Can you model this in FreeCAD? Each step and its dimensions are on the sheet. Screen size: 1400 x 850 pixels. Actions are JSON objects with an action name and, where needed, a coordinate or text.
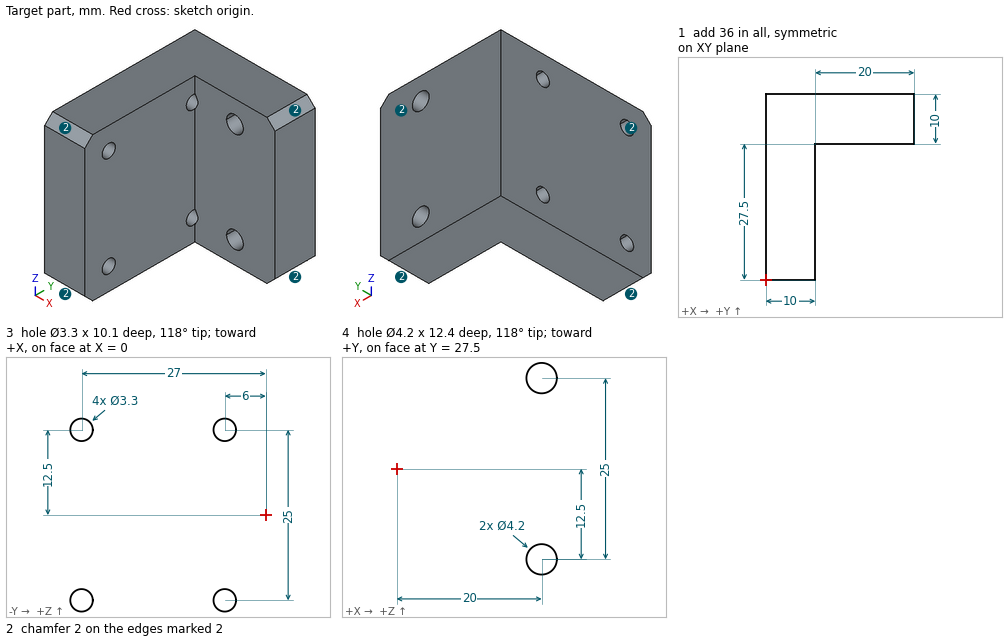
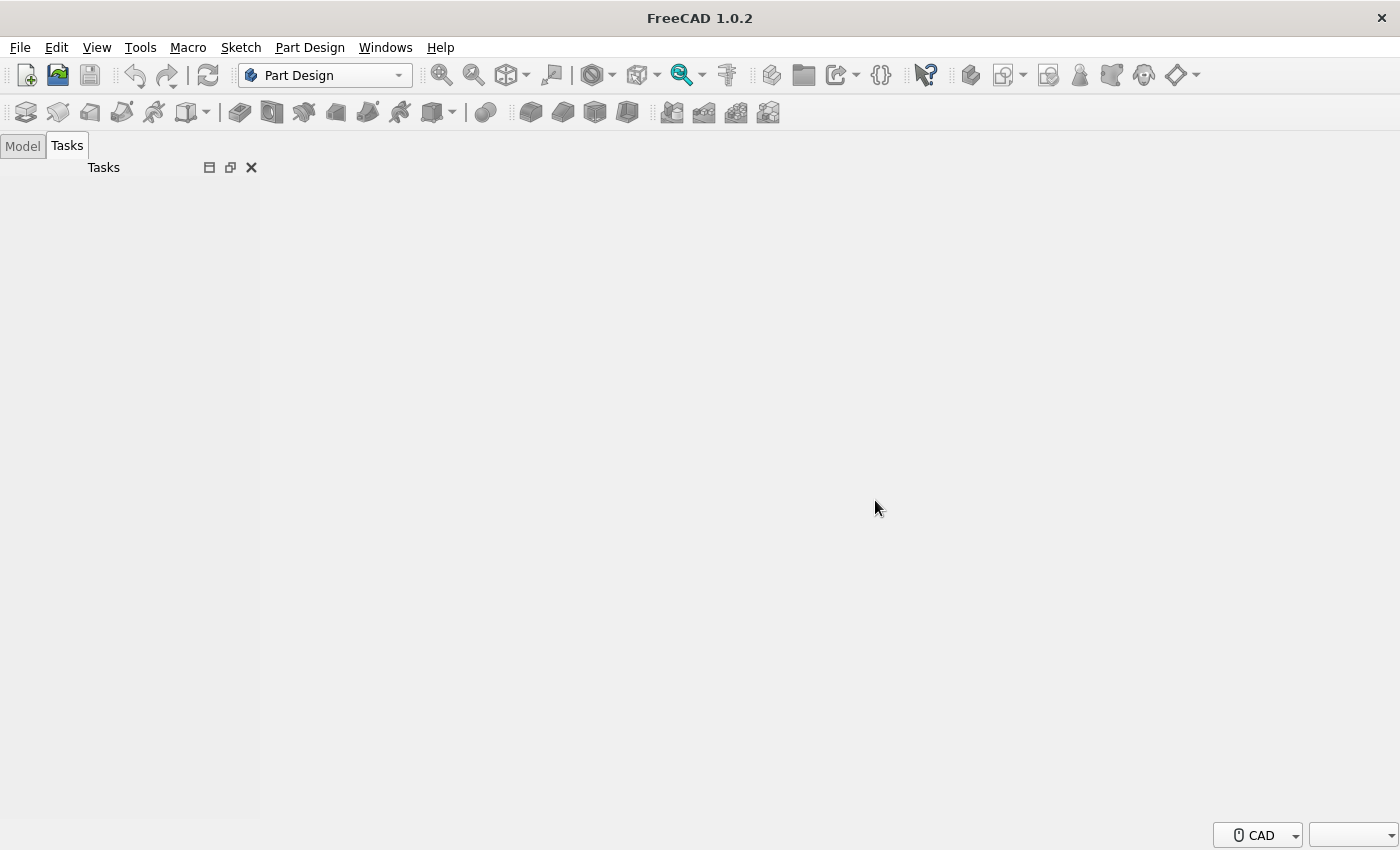
{"action": "key", "text": "ctrl+n"}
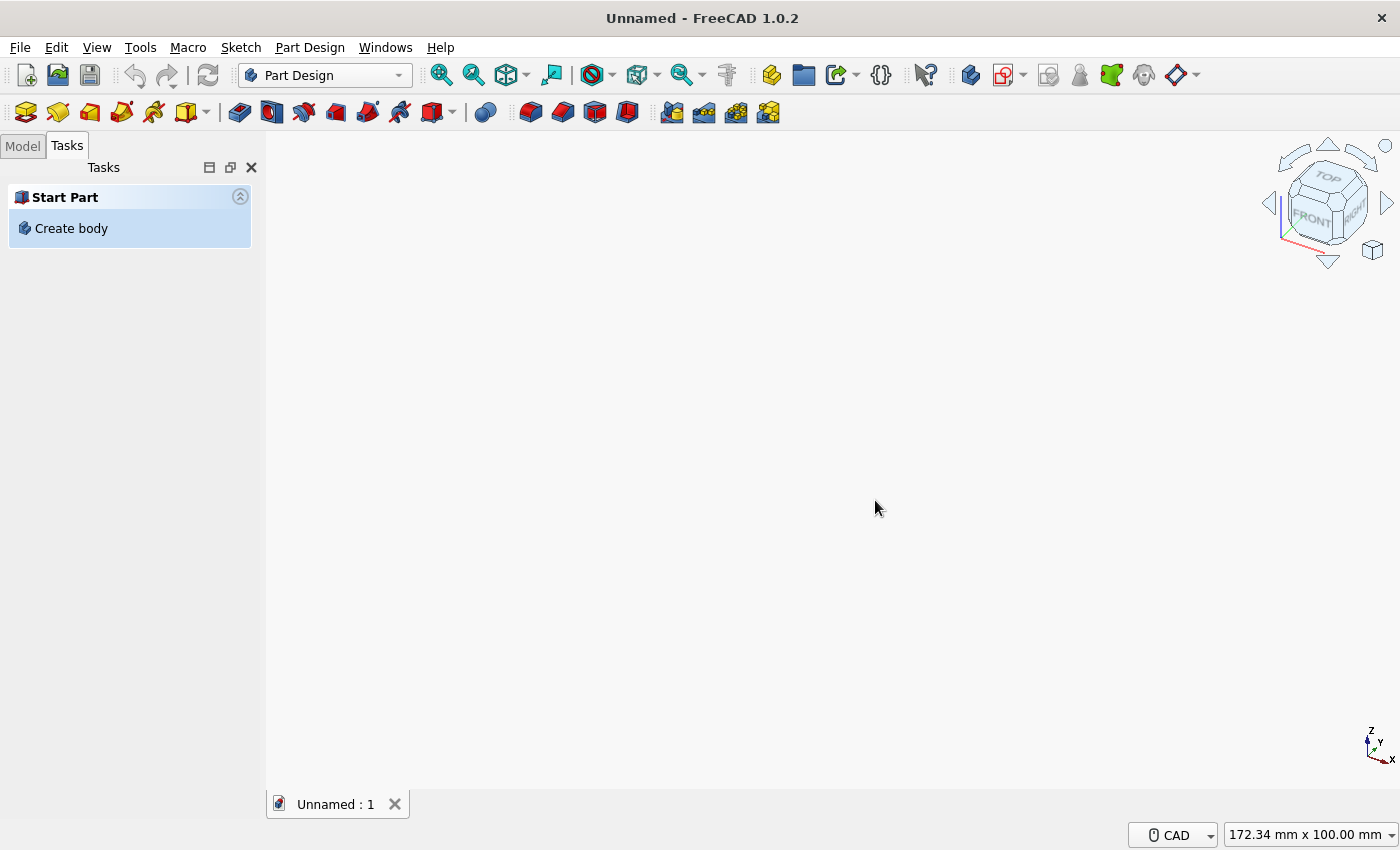
{"action": "left_click", "coordinate": [1004, 76]}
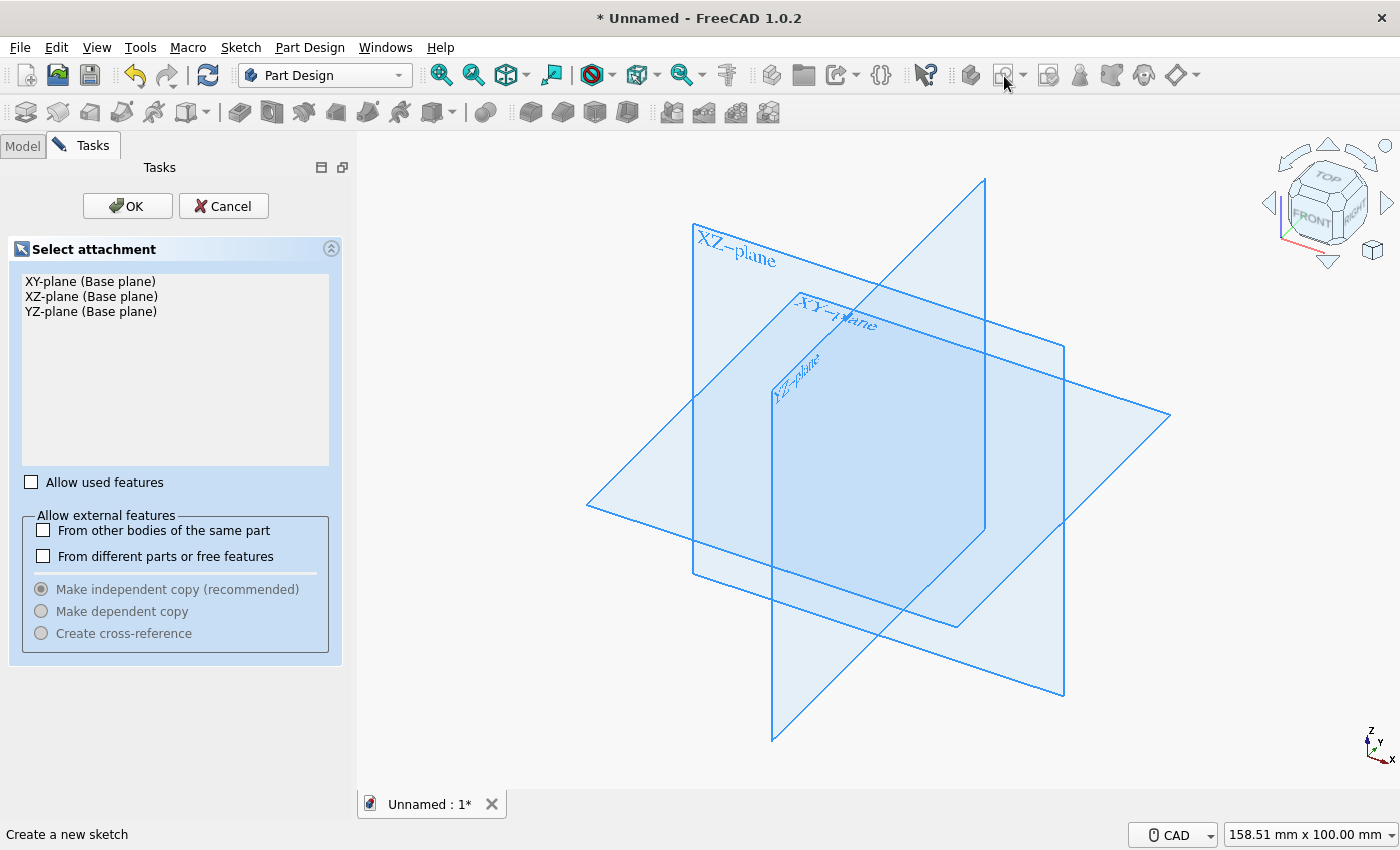
{"action": "left_click", "coordinate": [82, 282]}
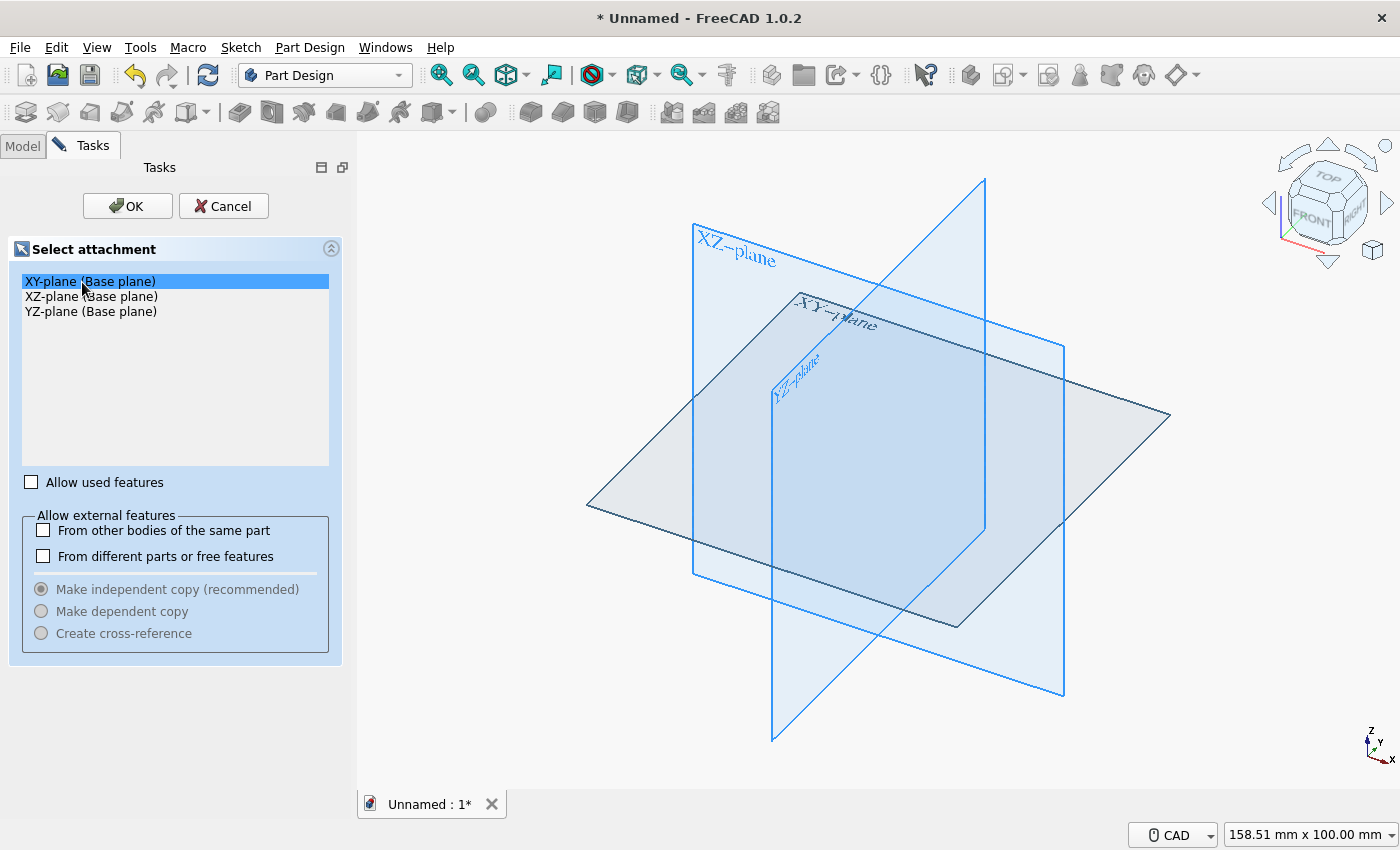
{"action": "left_click", "coordinate": [128, 206]}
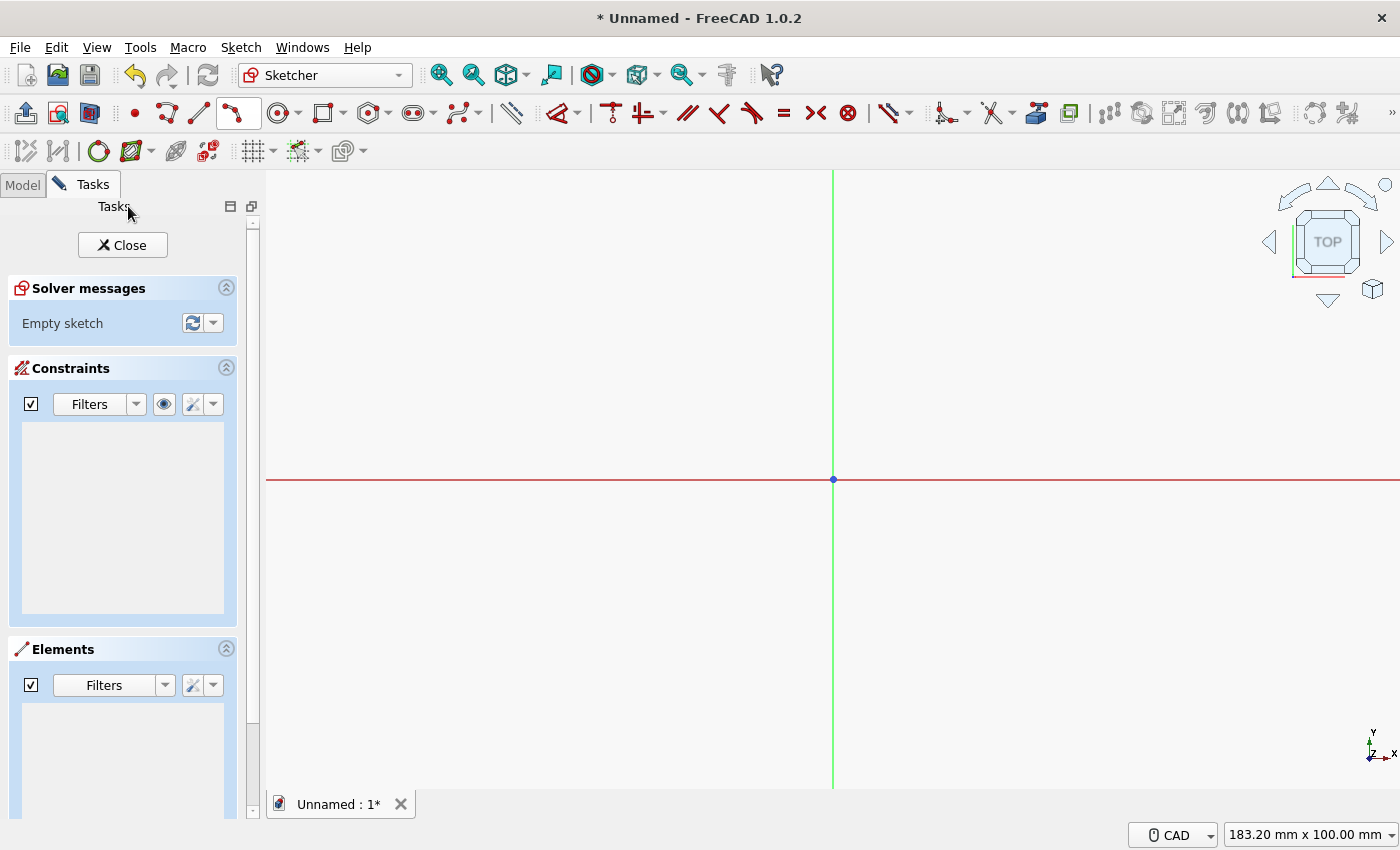
{"action": "scroll", "coordinate": [1122, 222], "scroll_direction": "up", "scroll_amount": 3}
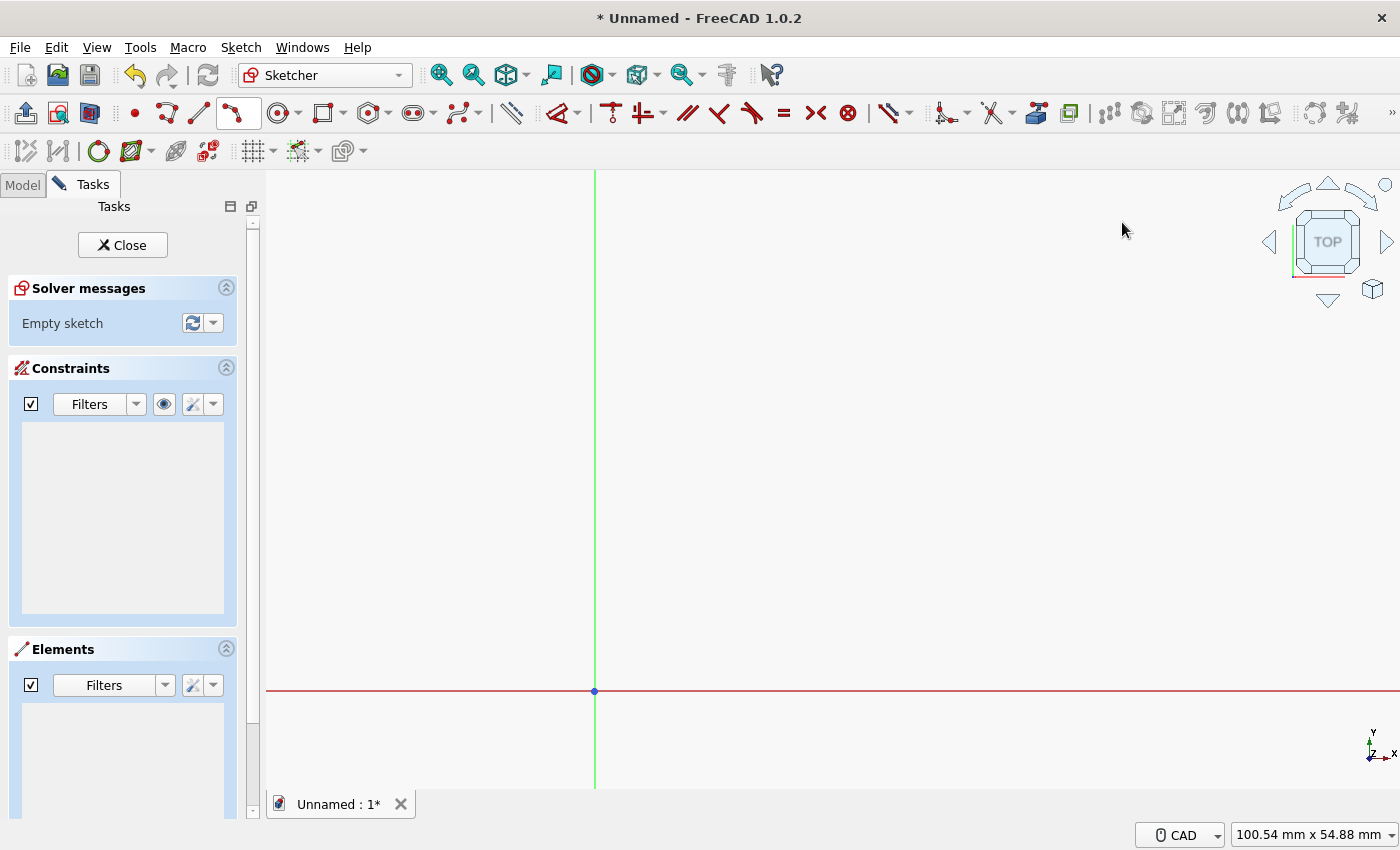
{"action": "key", "text": "g m"}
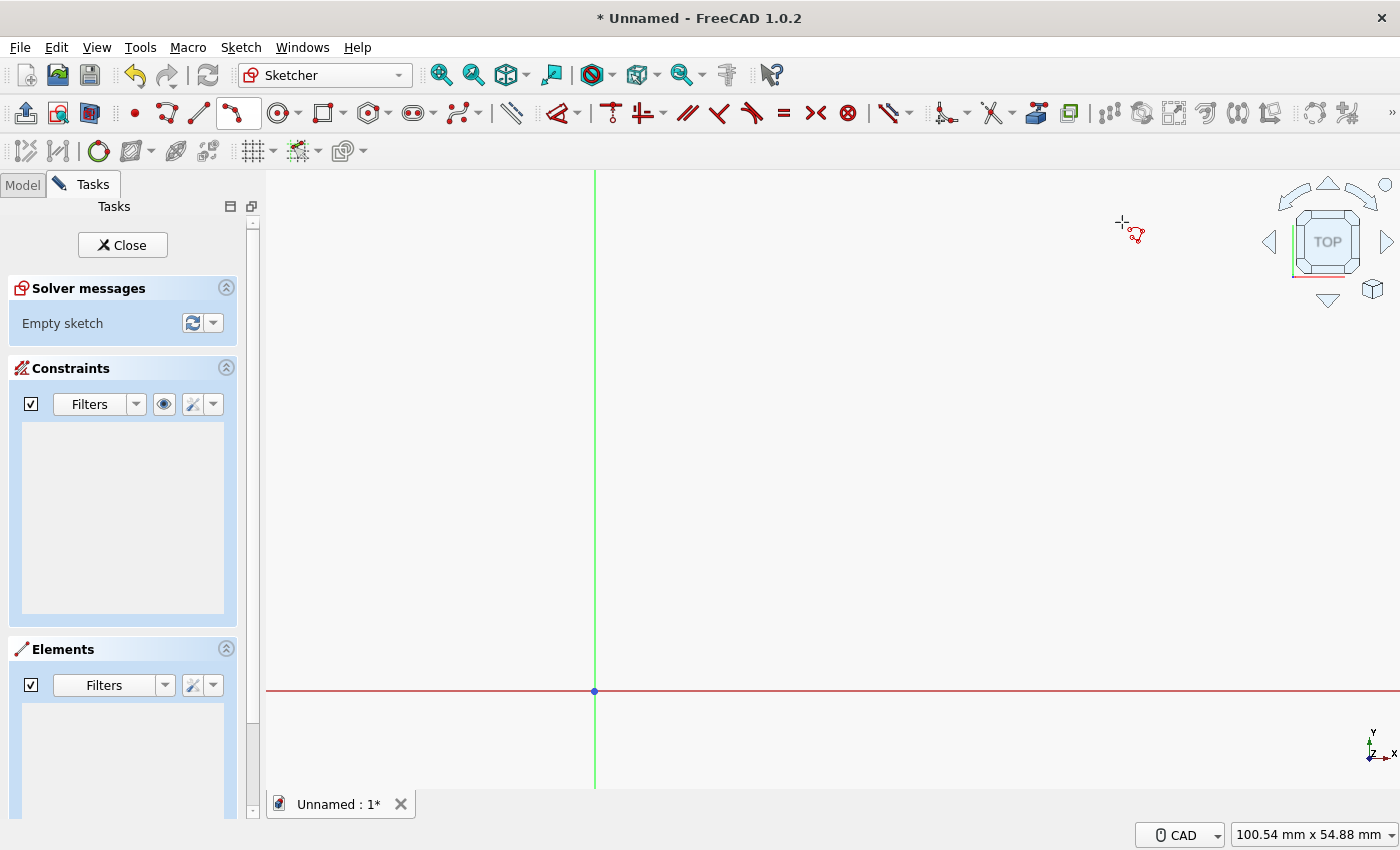
{"action": "left_click", "coordinate": [595, 691]}
{"action": "left_click", "coordinate": [708, 682]}
{"action": "left_click", "coordinate": [708, 381]}
{"action": "left_click", "coordinate": [933, 381]}
{"action": "left_click", "coordinate": [933, 268]}
{"action": "left_click", "coordinate": [604, 268]}
{"action": "left_click", "coordinate": [595, 691]}
{"action": "key", "text": "Escape"}
{"action": "key", "text": "Escape"}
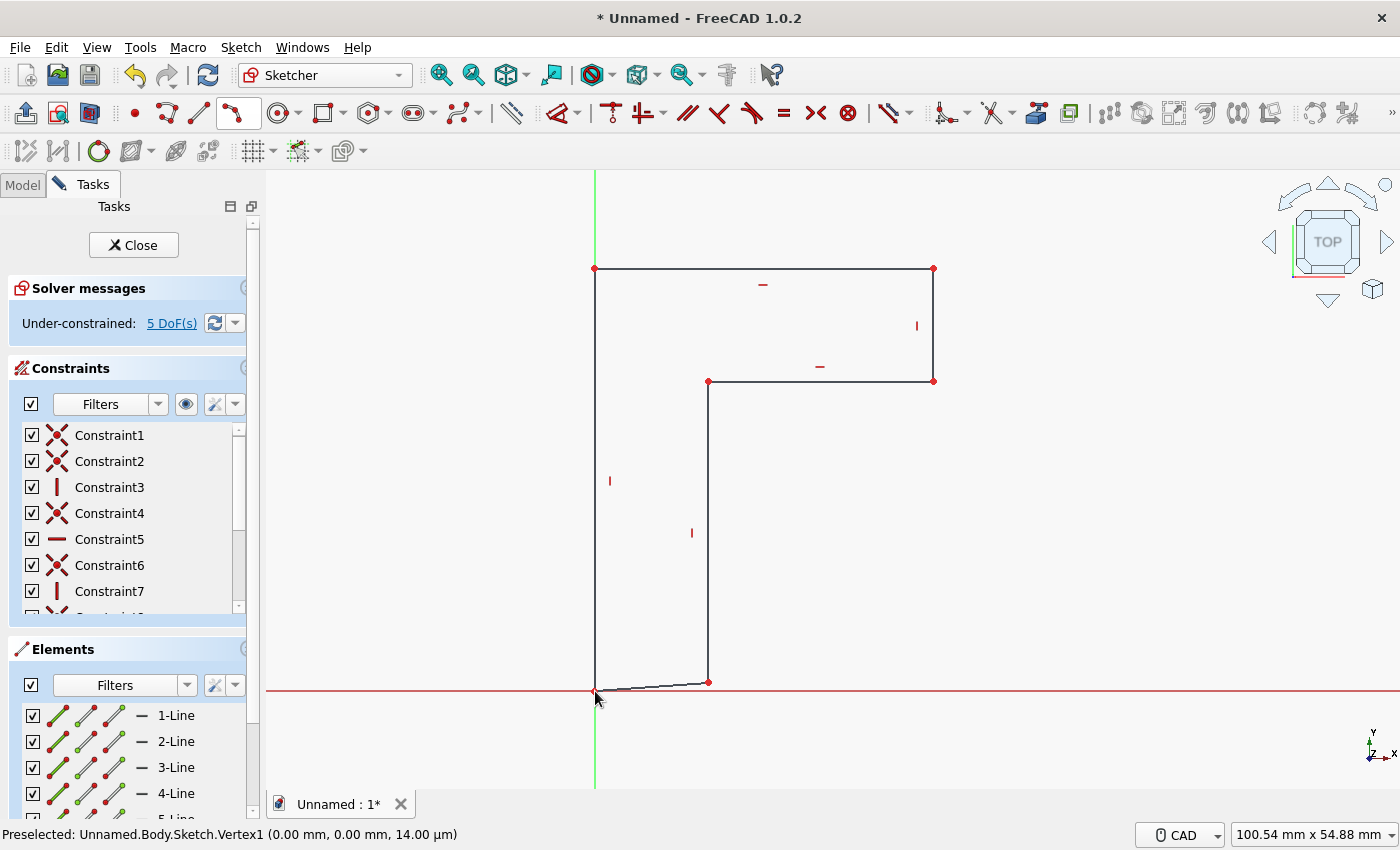
{"action": "left_click", "coordinate": [629, 689]}